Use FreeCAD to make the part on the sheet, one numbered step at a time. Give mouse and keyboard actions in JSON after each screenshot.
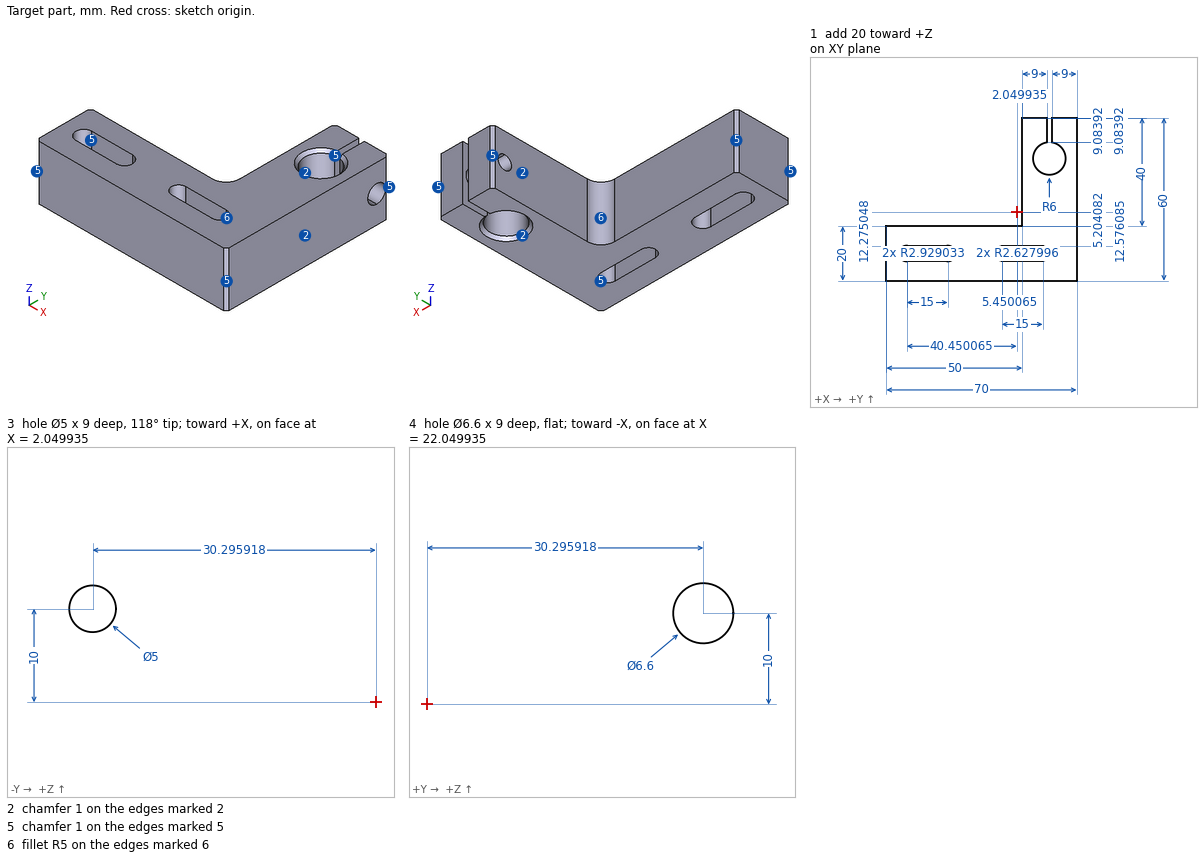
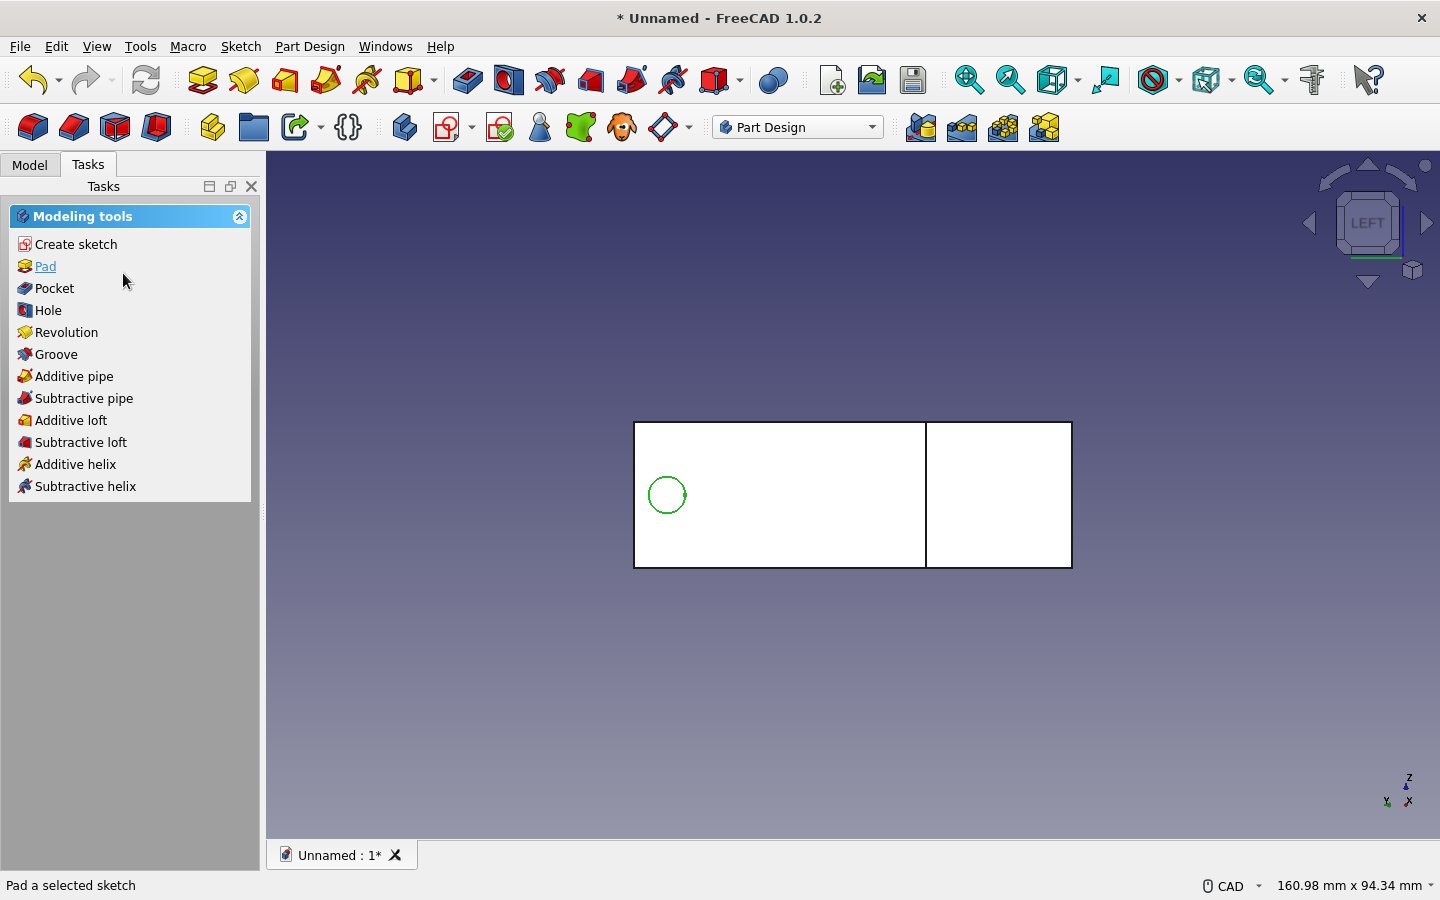
{"action": "left_click", "coordinate": [509, 80]}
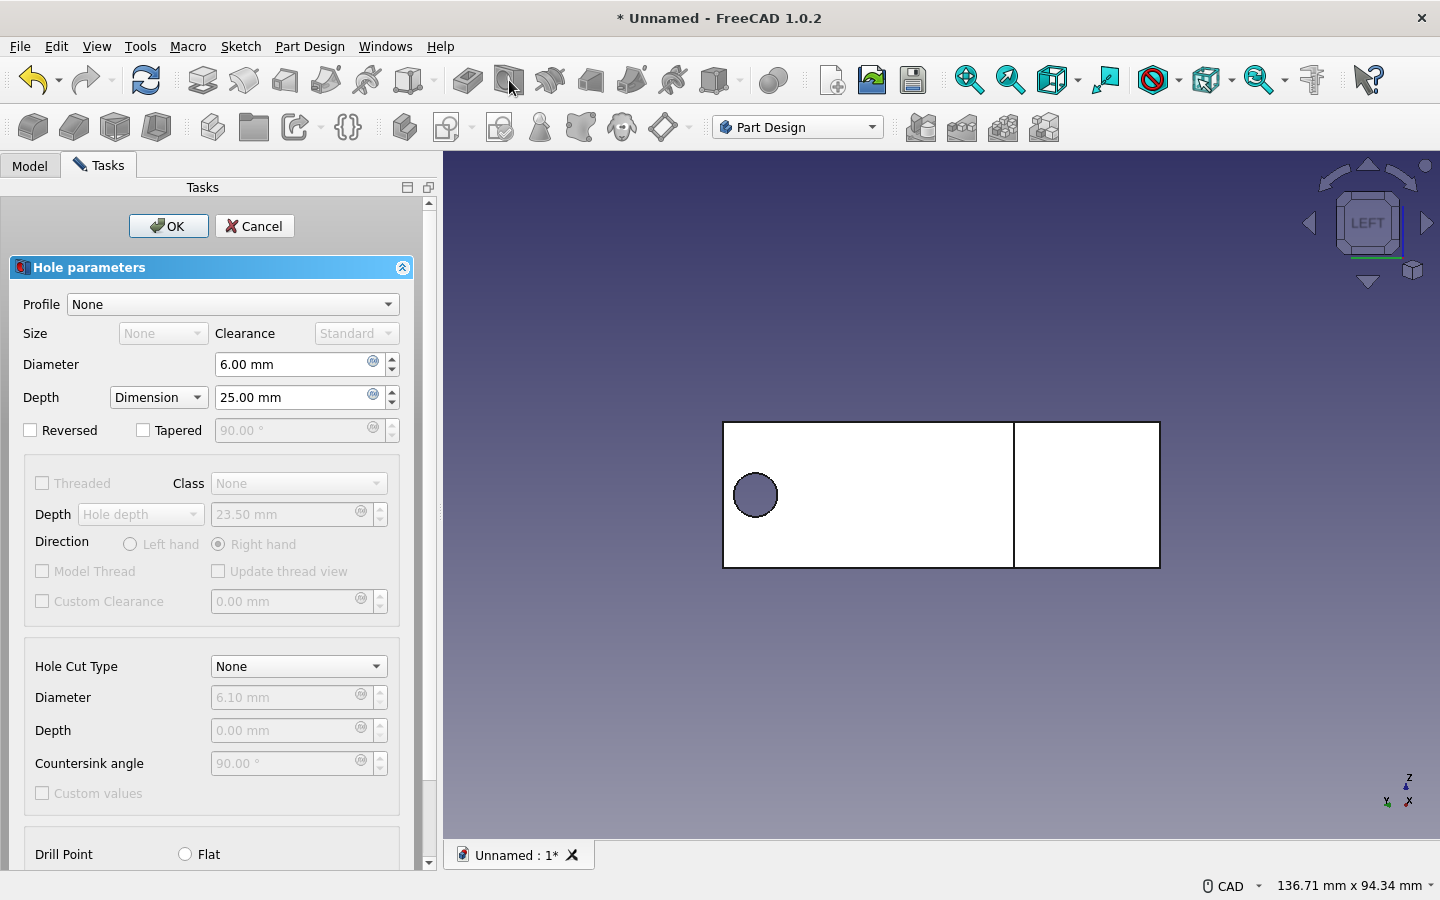
{"action": "triple_click", "coordinate": [300, 364]}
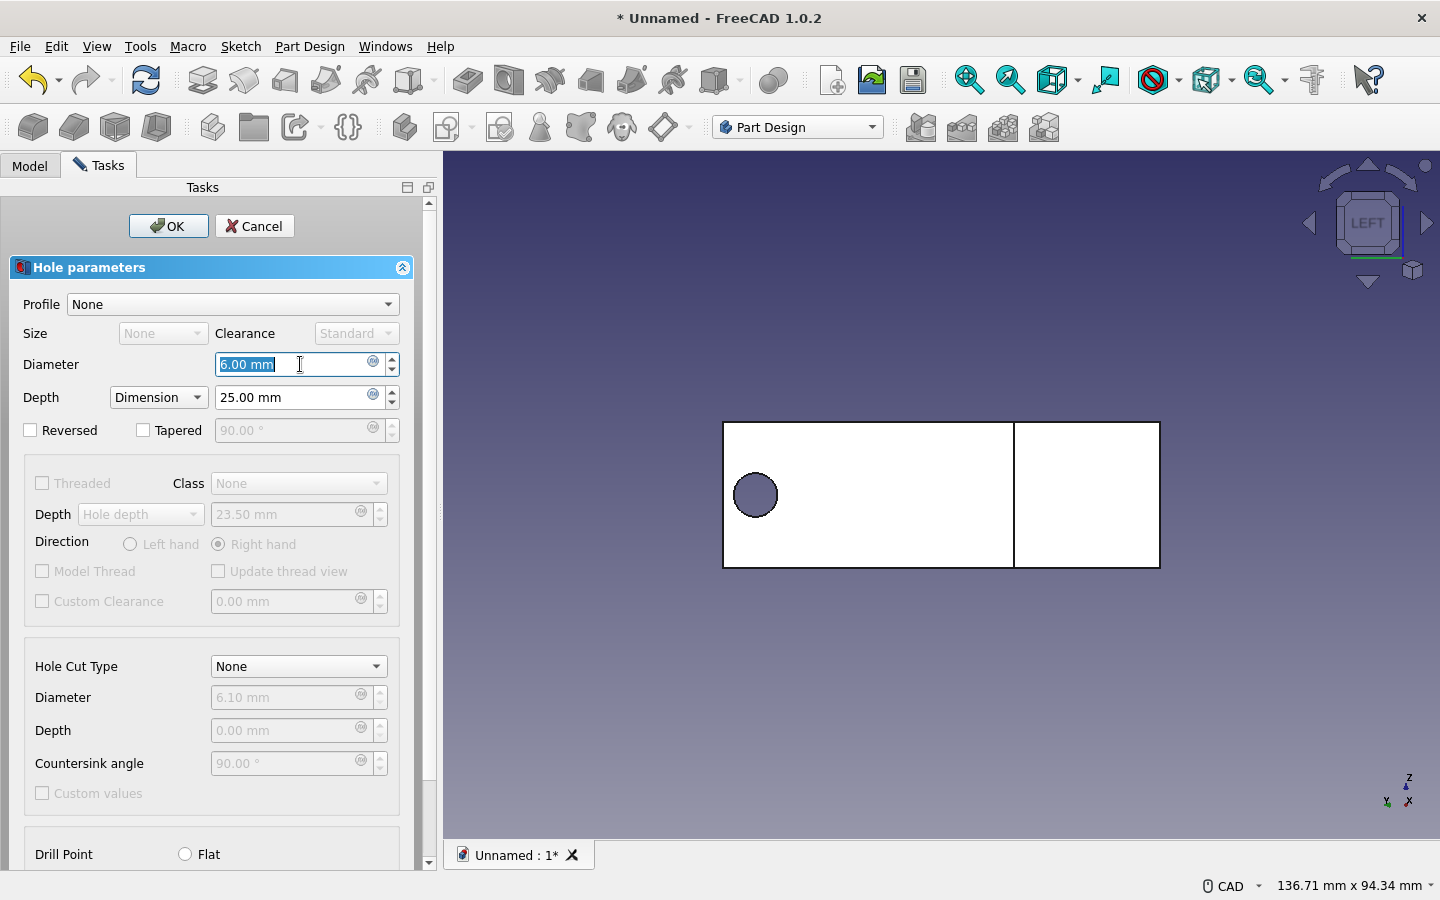
{"action": "type", "text": "5"}
{"action": "key", "text": "Tab"}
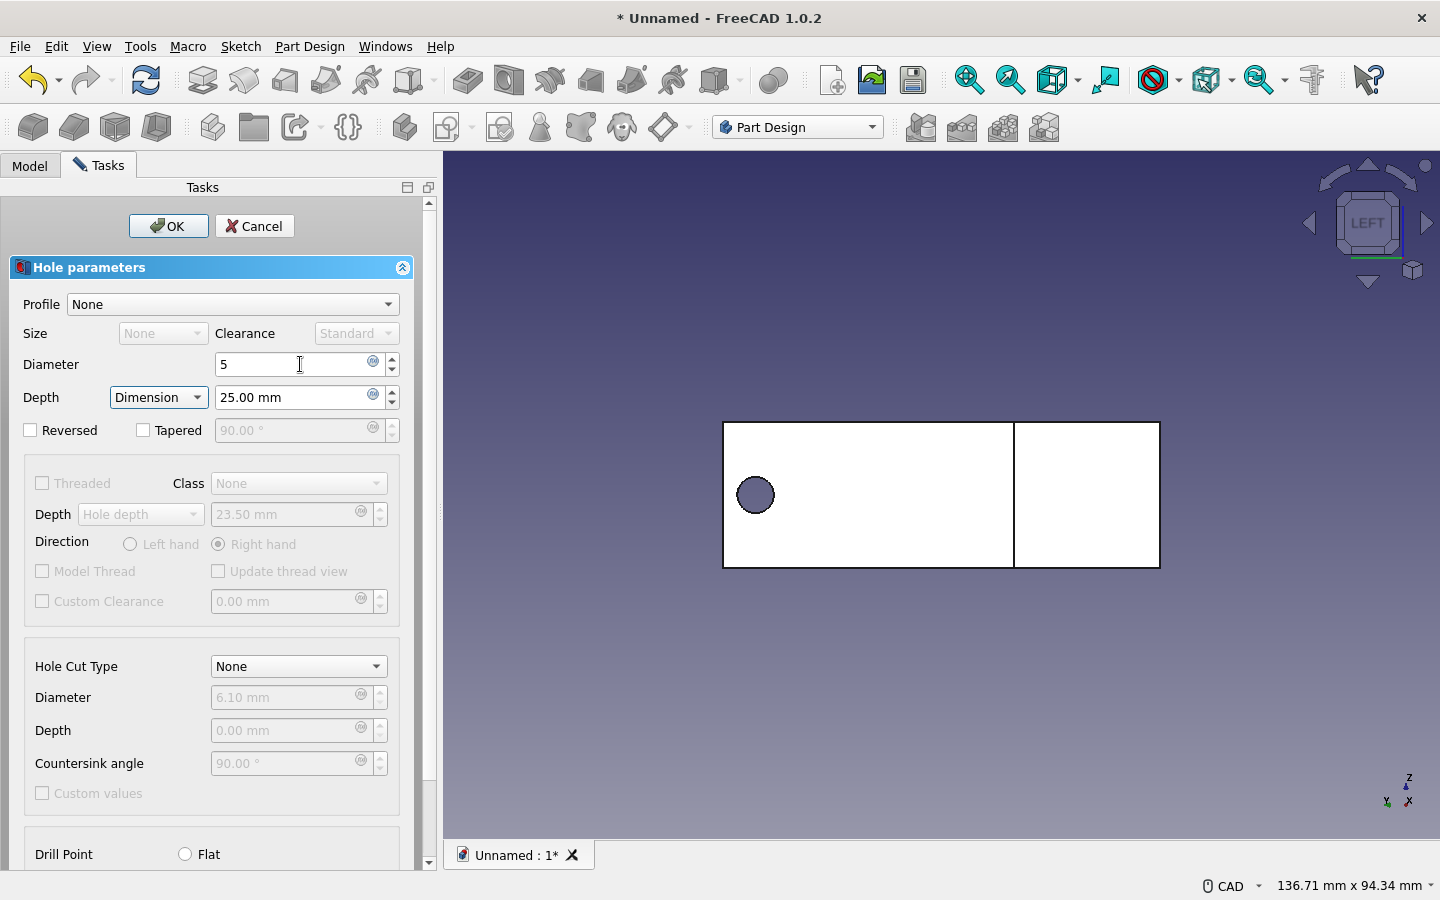
{"action": "triple_click", "coordinate": [300, 398]}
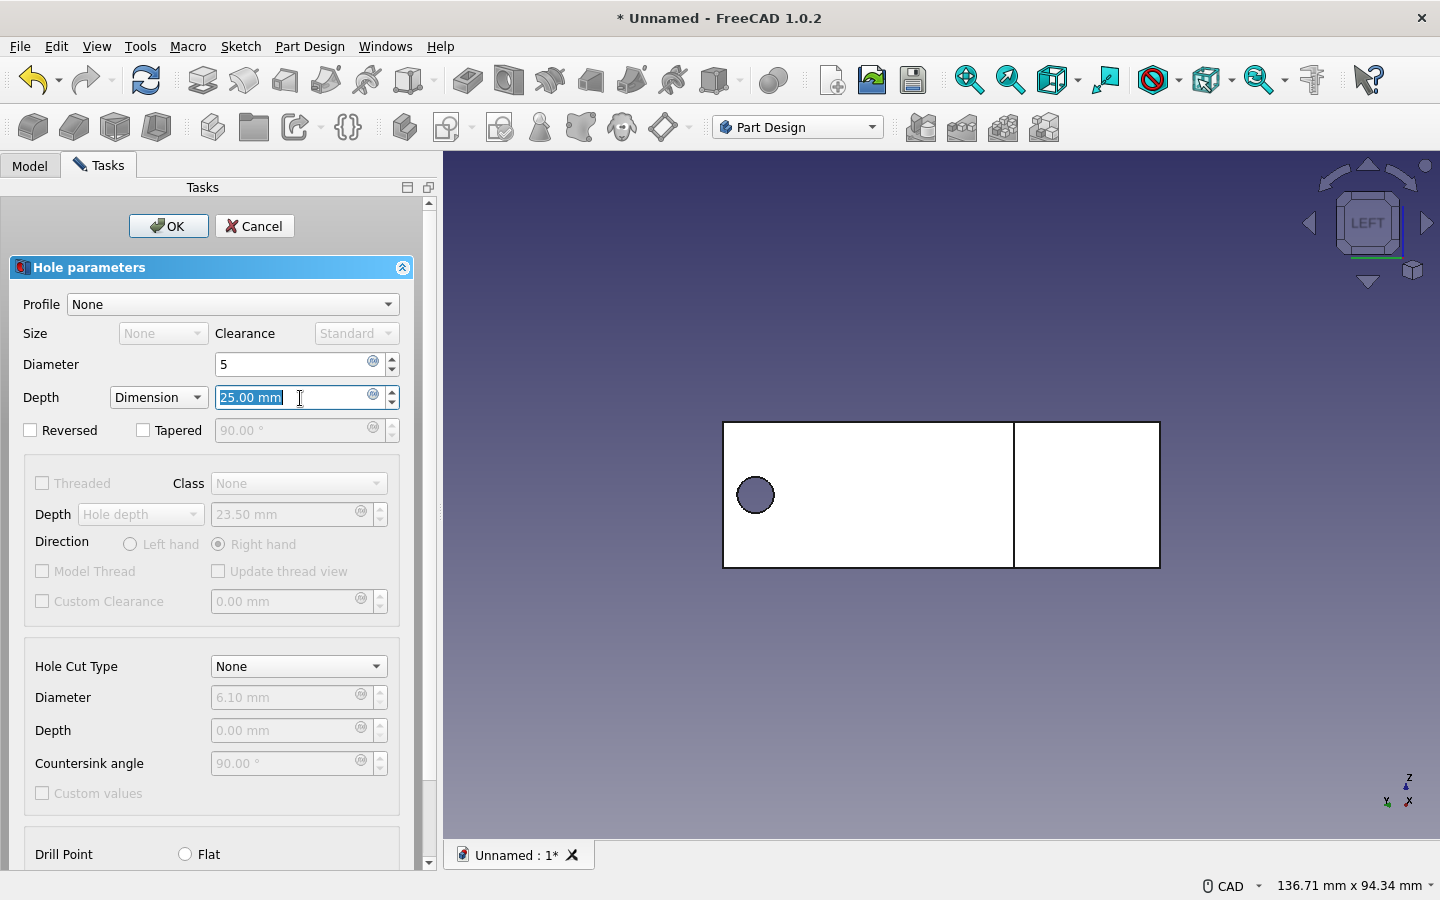
{"action": "type", "text": "9"}
{"action": "key", "text": "Tab"}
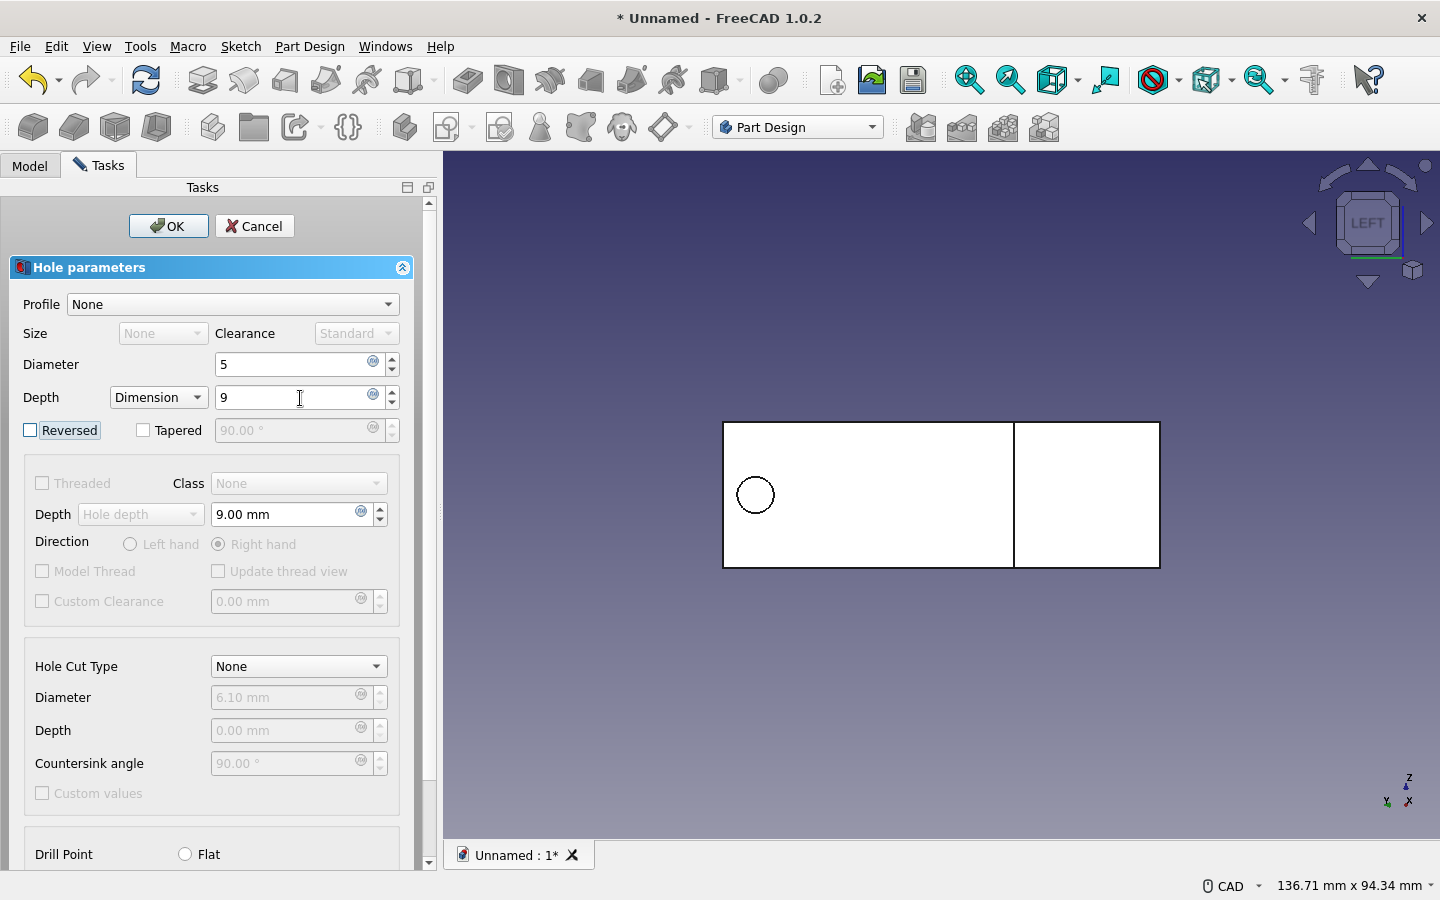
{"action": "left_click", "coordinate": [169, 226]}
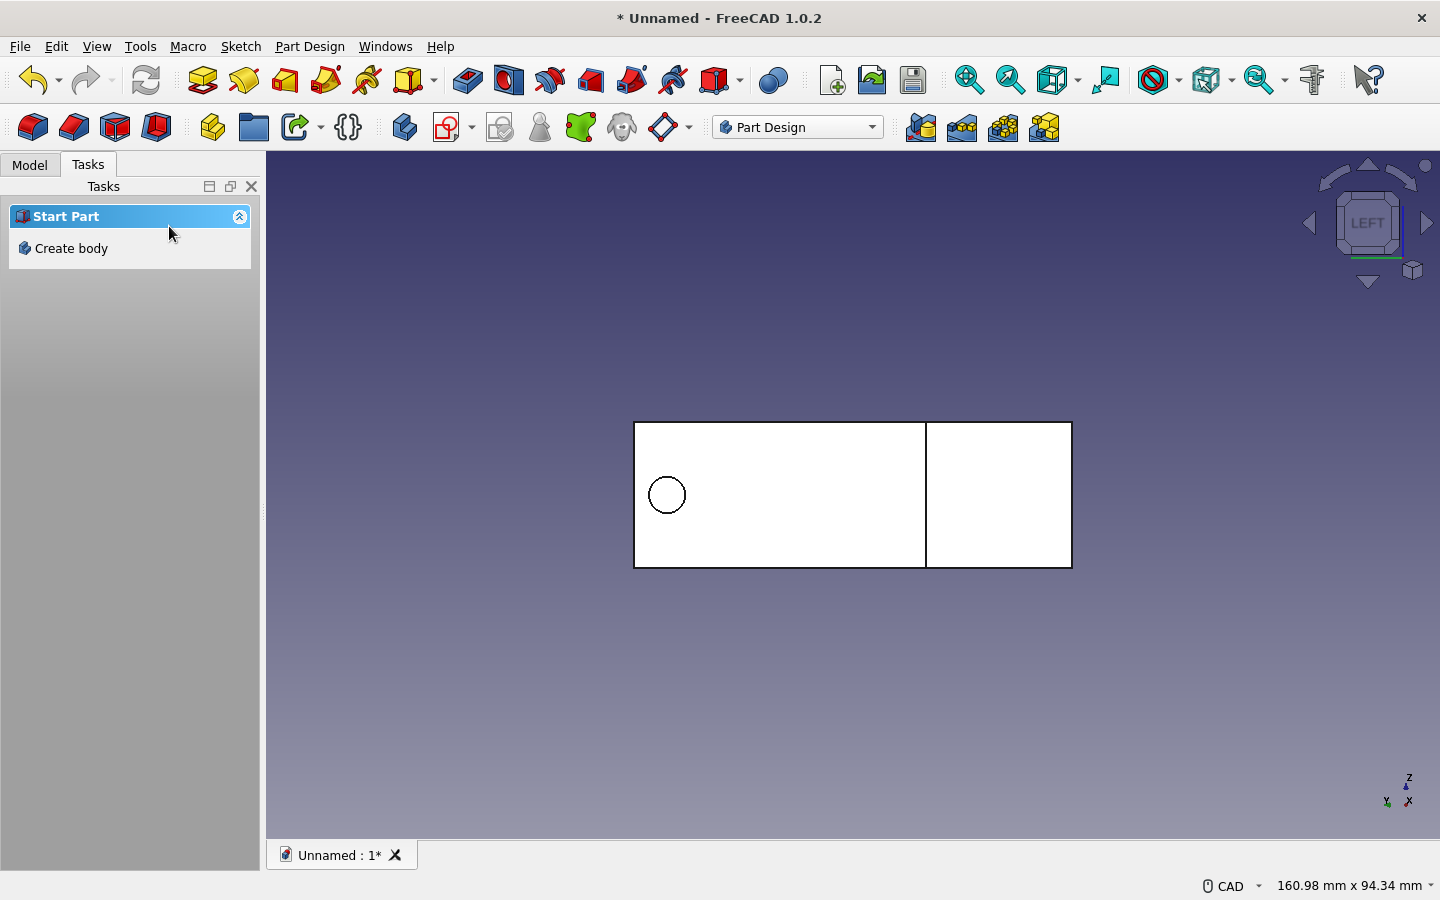
{"action": "left_click", "coordinate": [970, 80]}